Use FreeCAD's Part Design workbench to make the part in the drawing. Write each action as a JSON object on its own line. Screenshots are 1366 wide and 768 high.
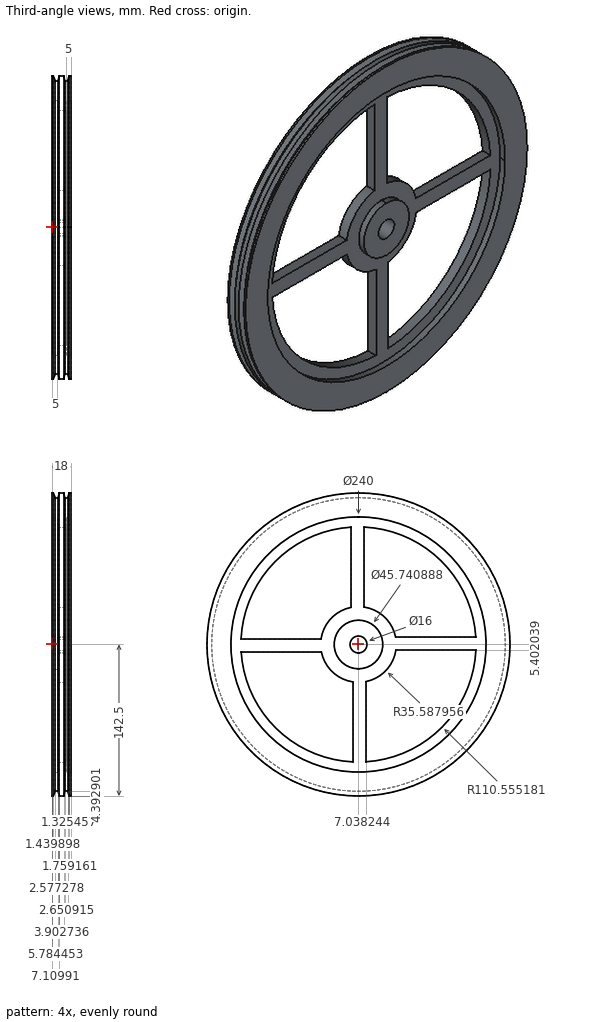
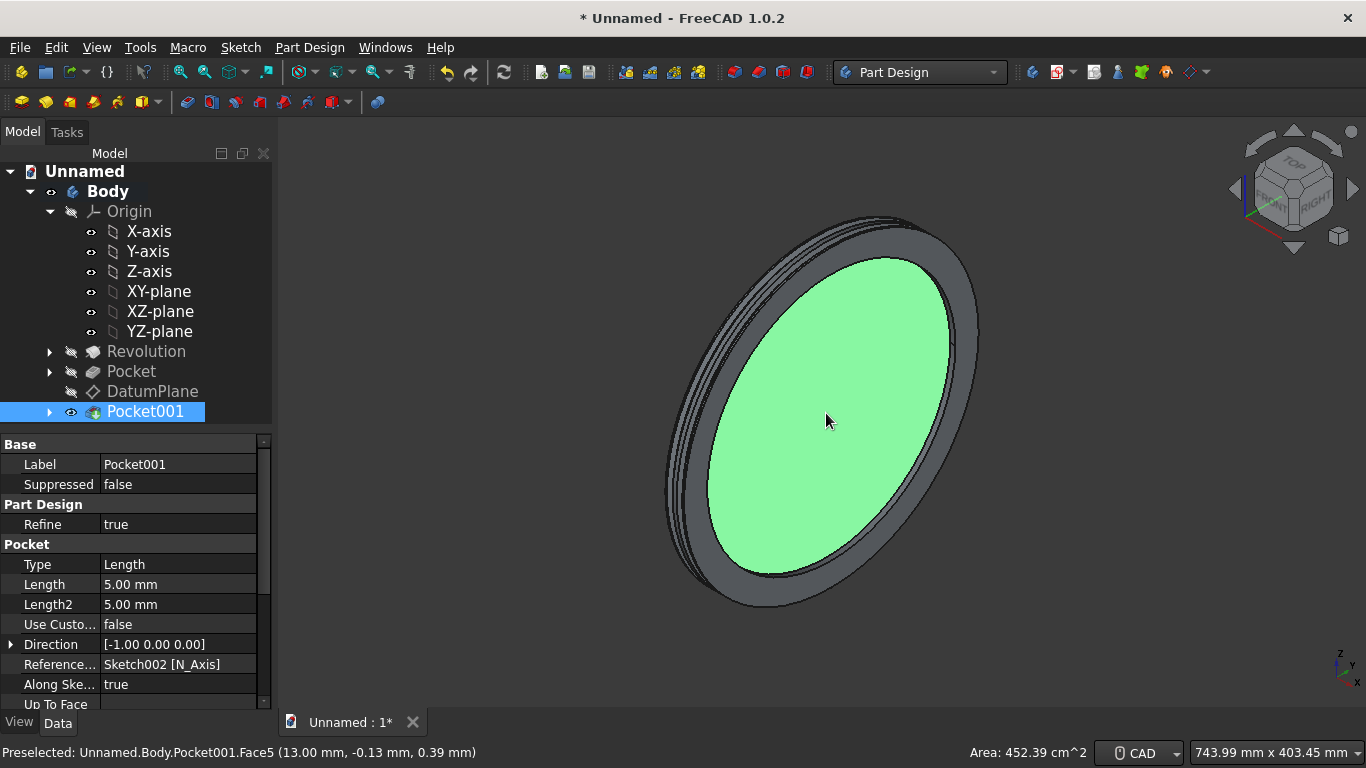
{"action": "left_click", "coordinate": [1058, 72]}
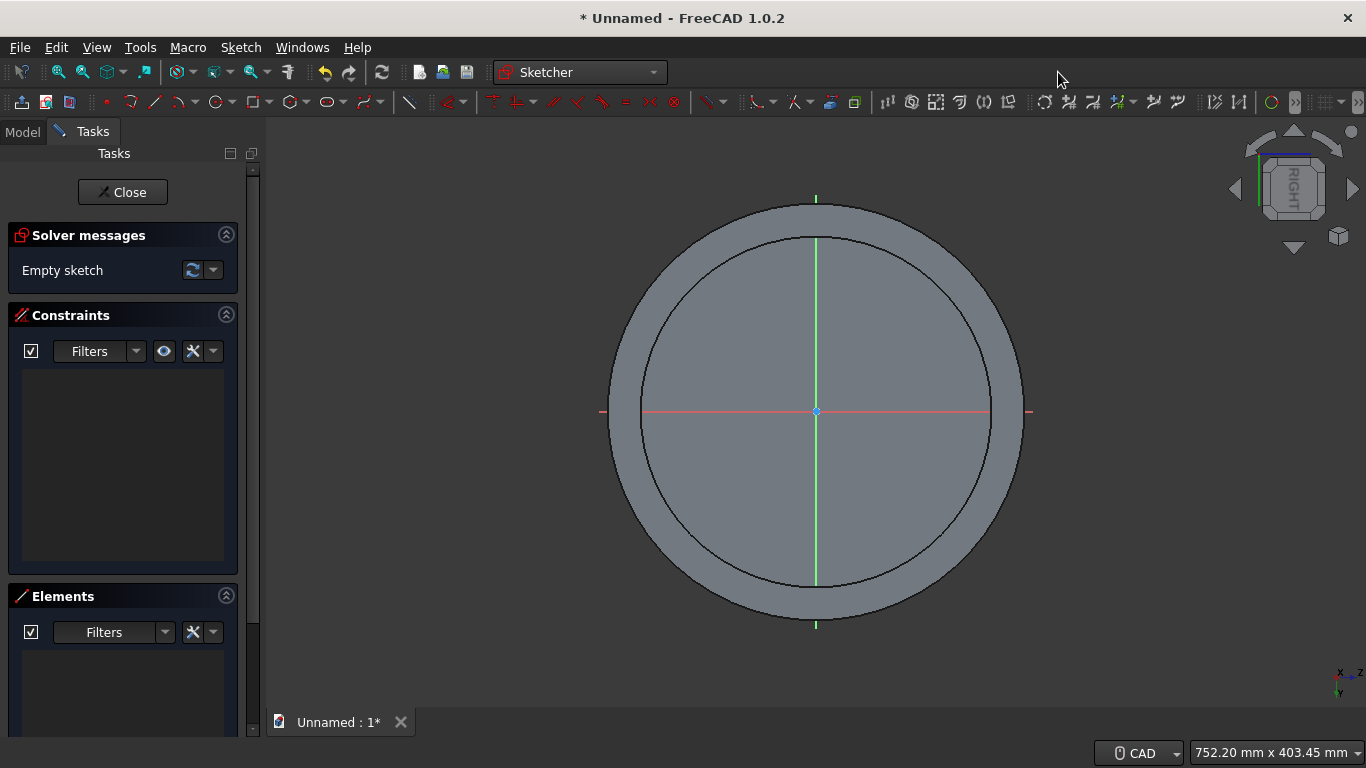
{"action": "scroll", "coordinate": [820, 412], "scroll_direction": "up", "scroll_amount": 14}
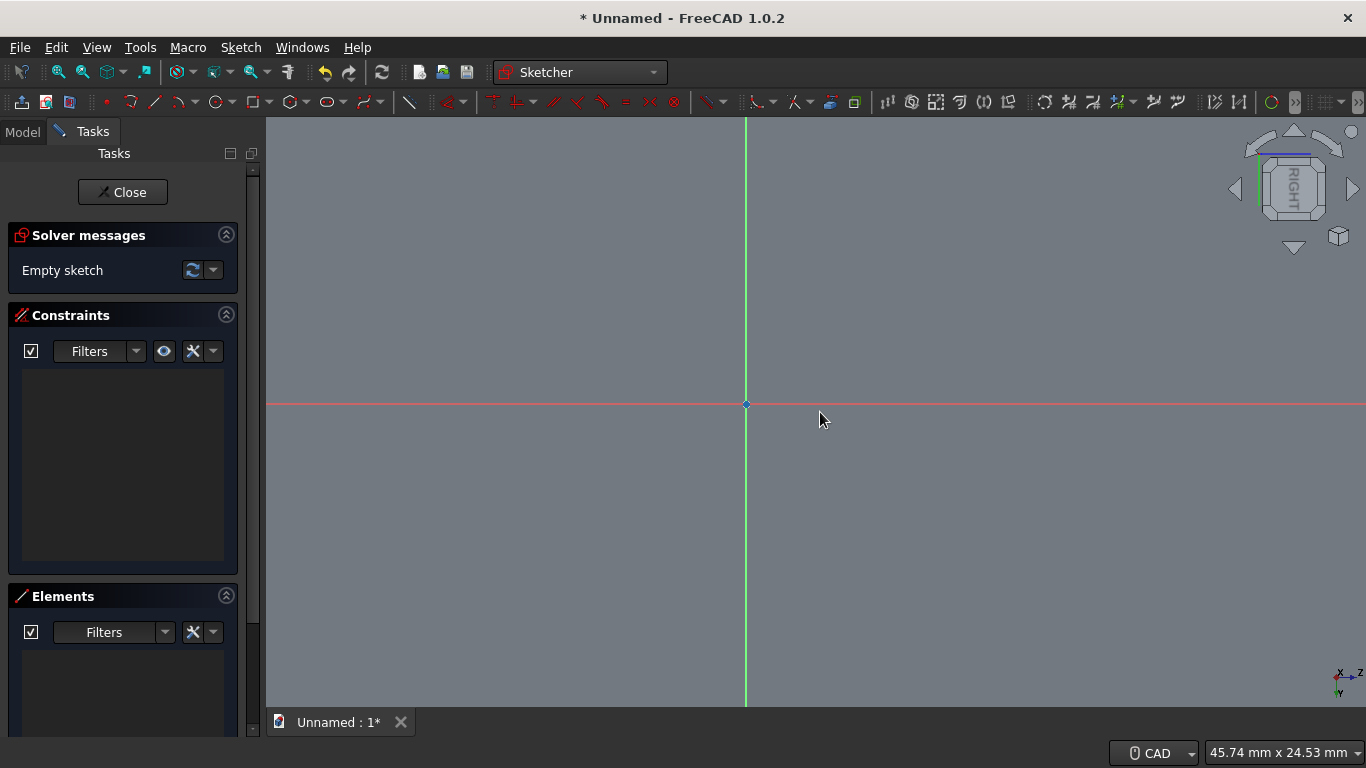
{"action": "key", "text": "g c"}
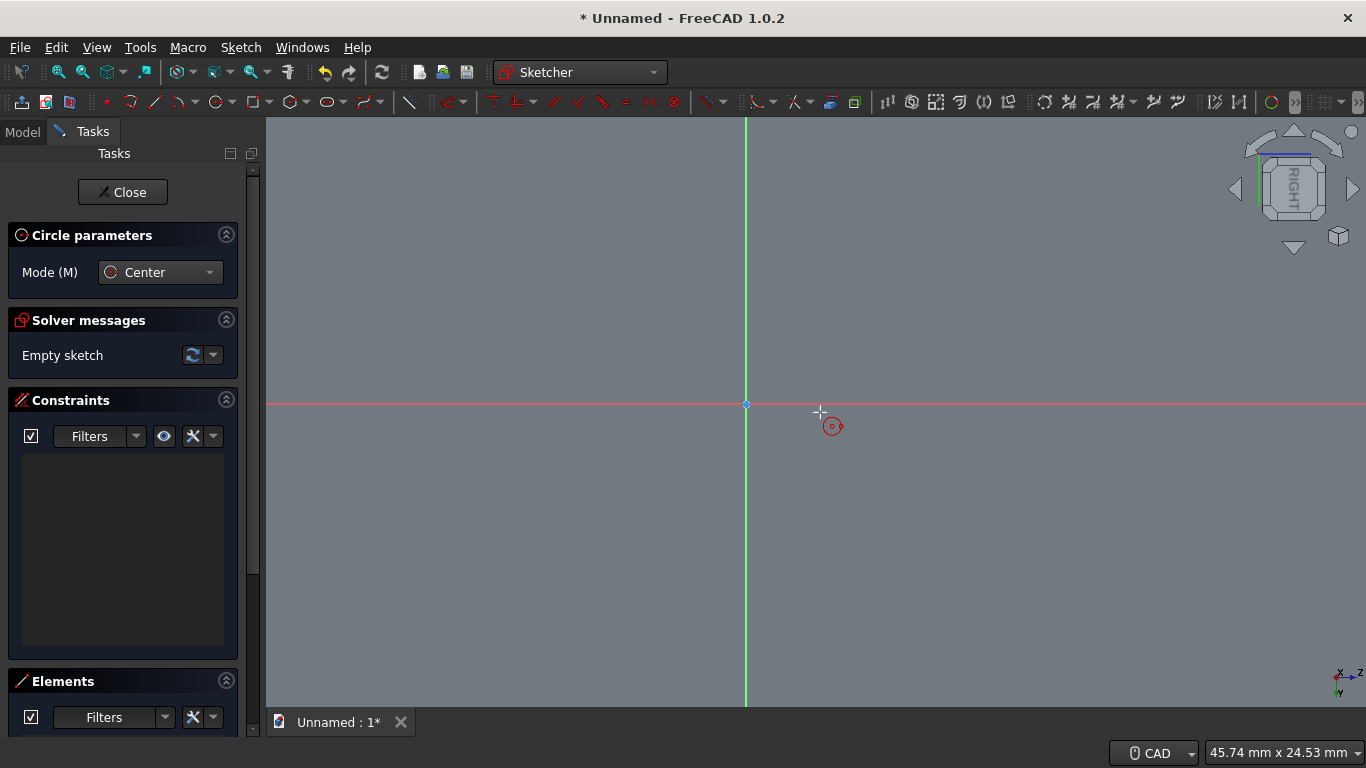
{"action": "left_click", "coordinate": [746, 404]}
{"action": "mouse_move", "coordinate": [882, 268]}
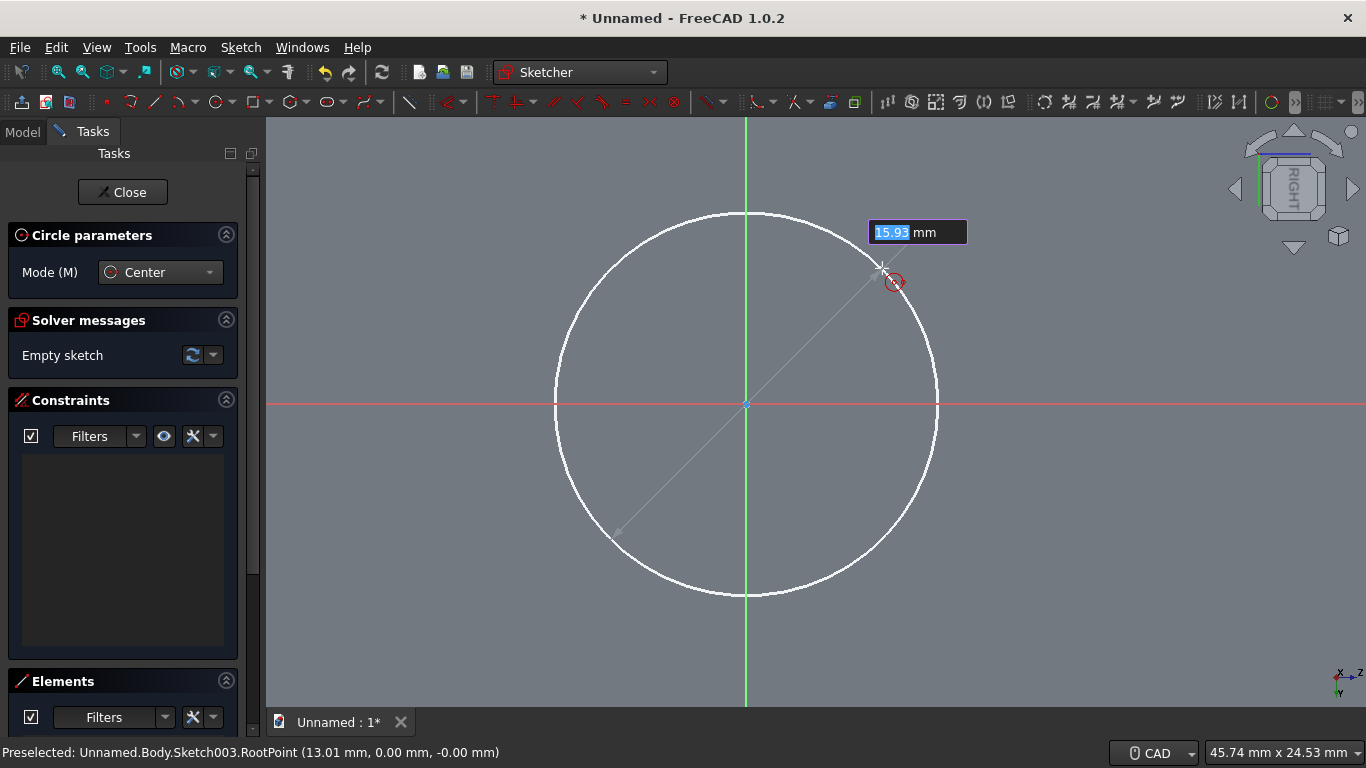
{"action": "type", "text": "16"}
{"action": "key", "text": "Return"}
{"action": "key", "text": "Escape"}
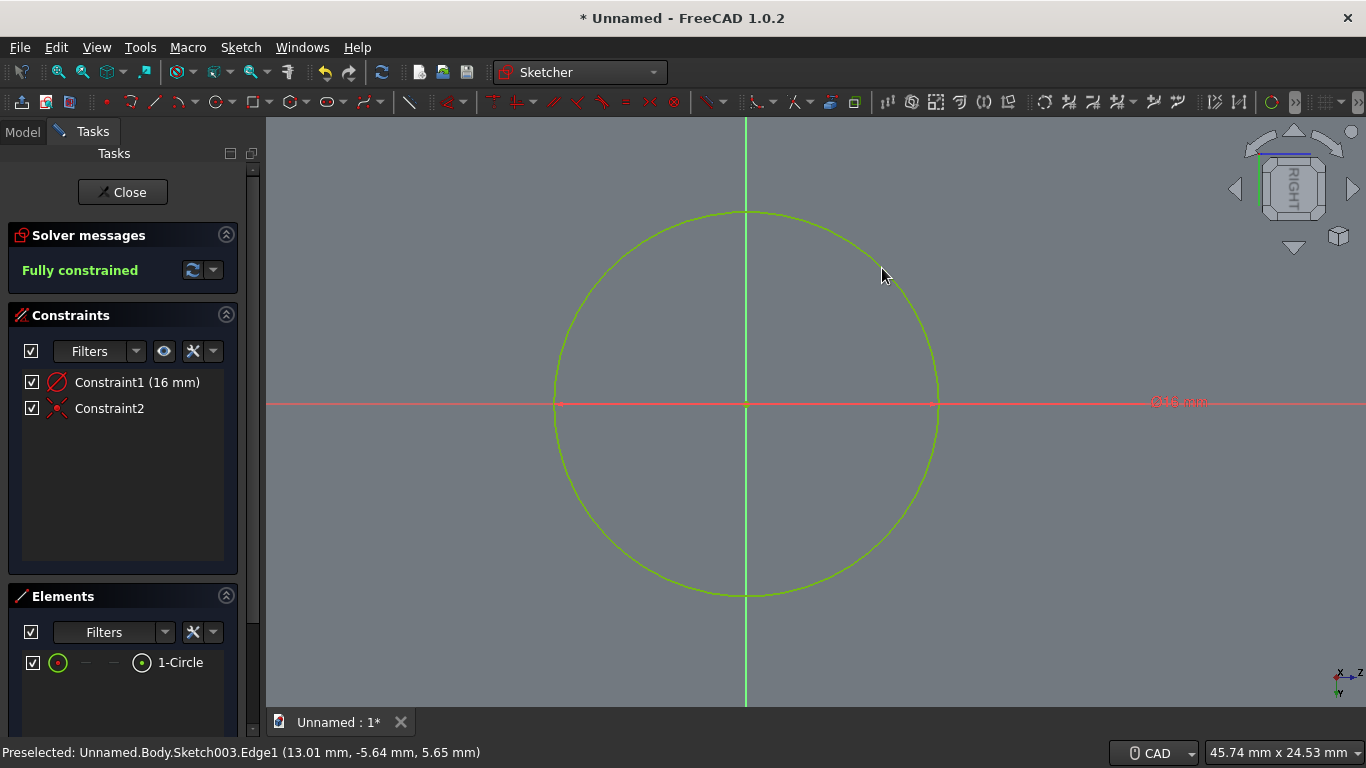
{"action": "left_click", "coordinate": [123, 192]}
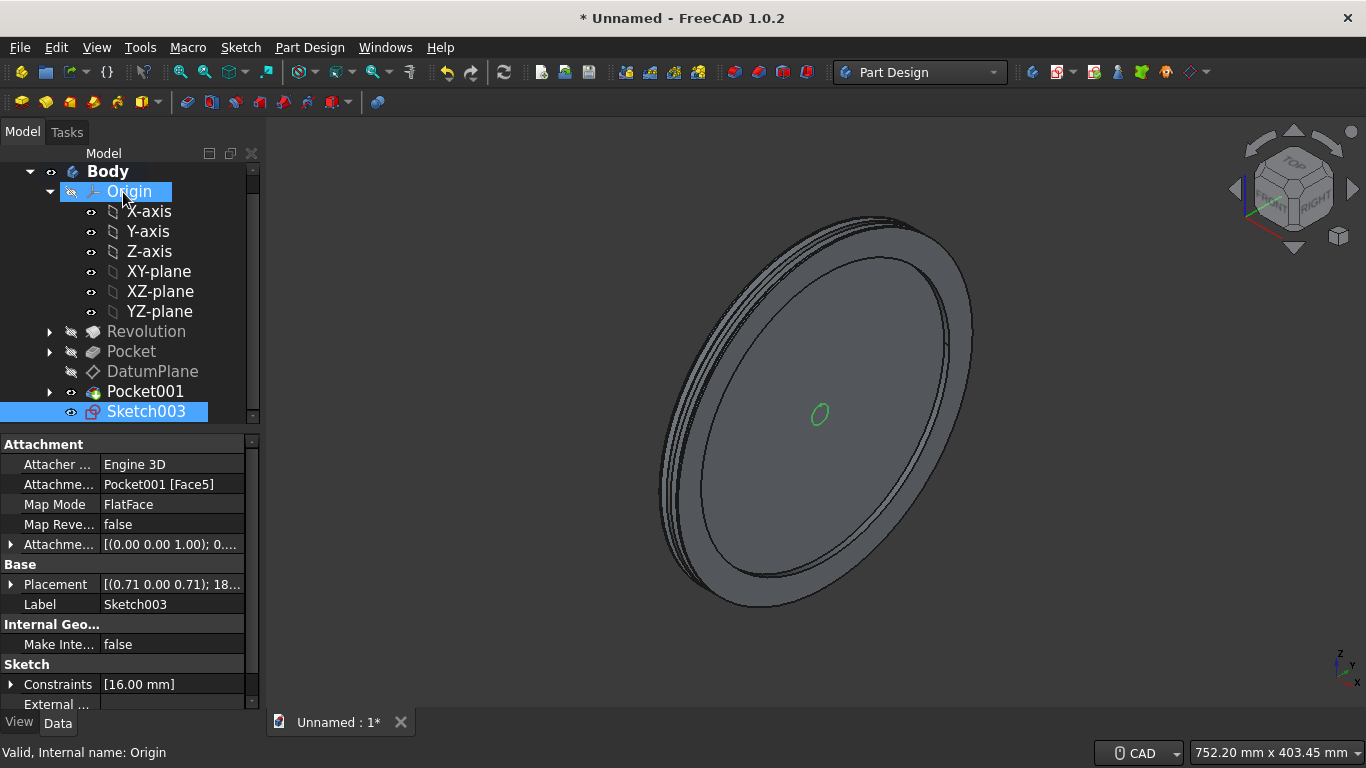
{"action": "left_click", "coordinate": [188, 102]}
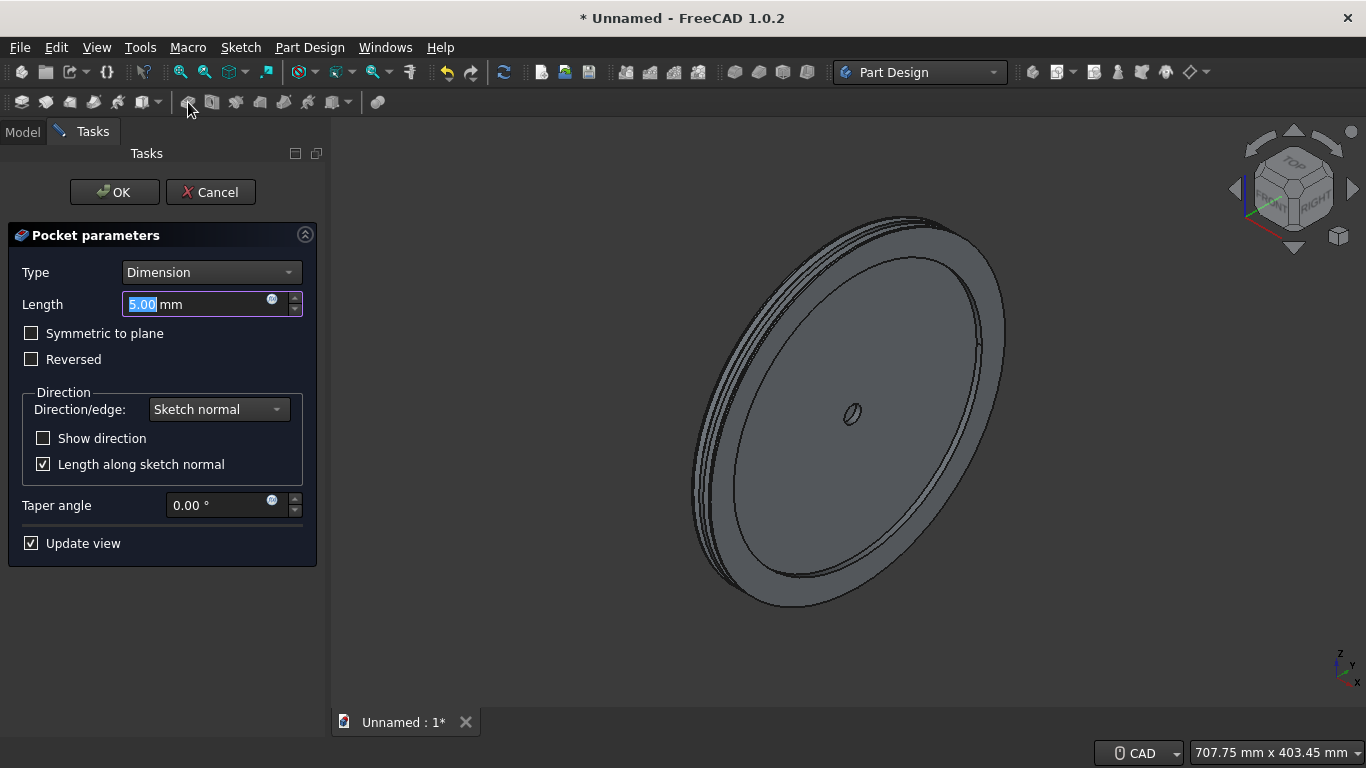
{"action": "left_click", "coordinate": [212, 272]}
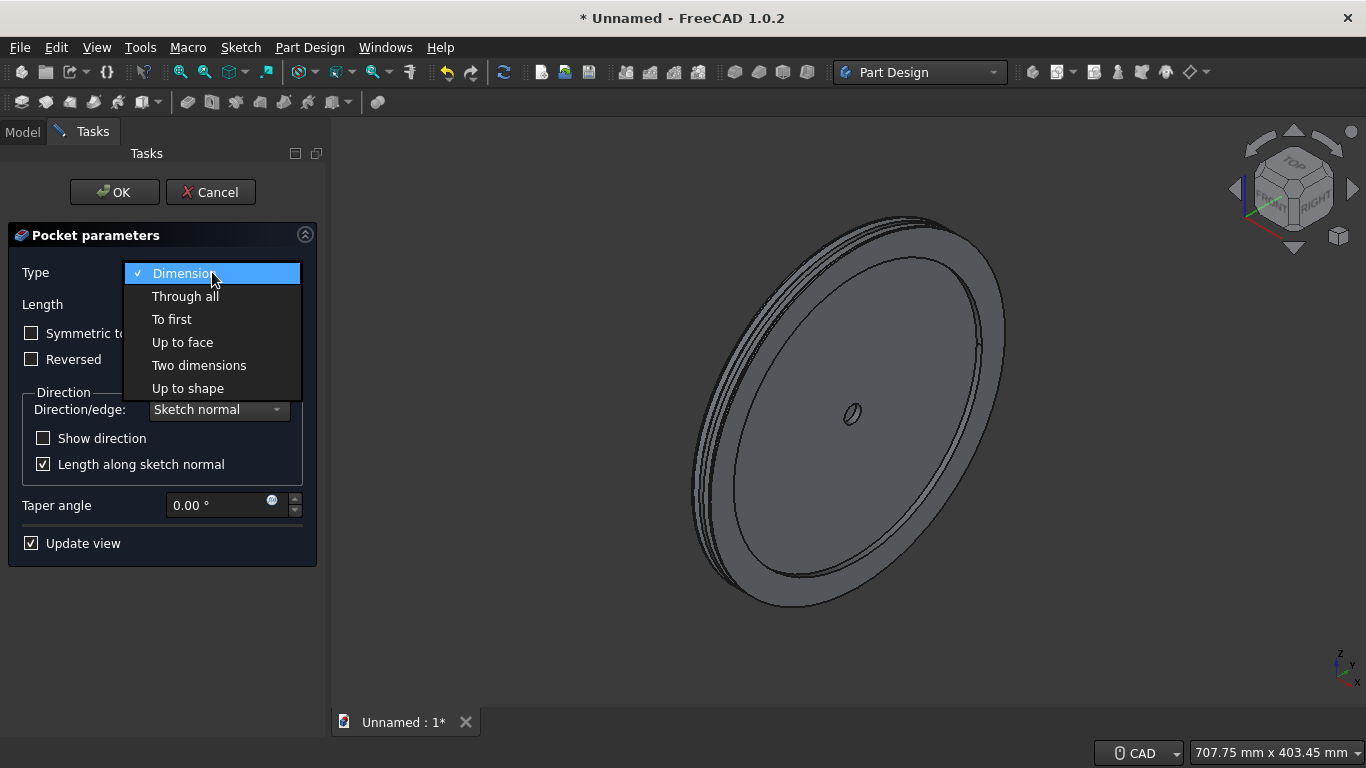
{"action": "left_click", "coordinate": [212, 296]}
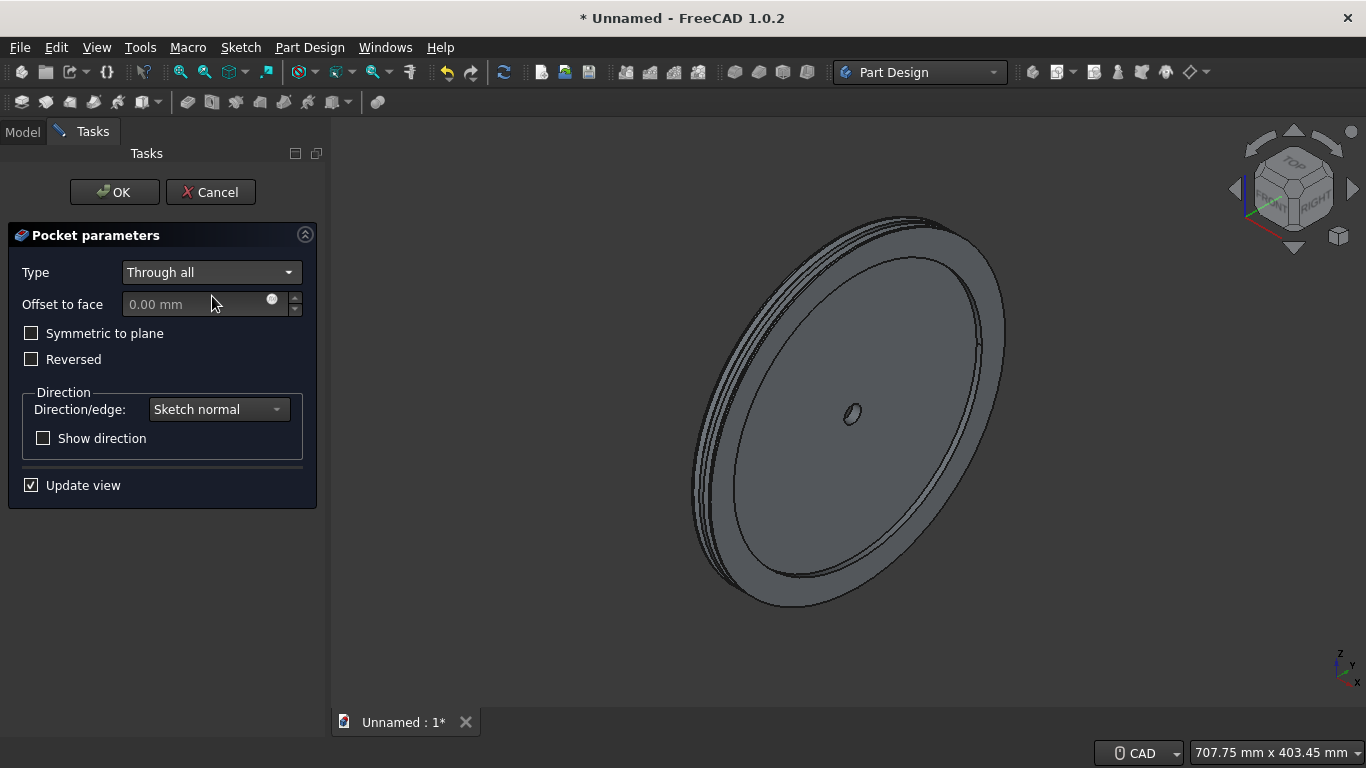
{"action": "left_click", "coordinate": [115, 192]}